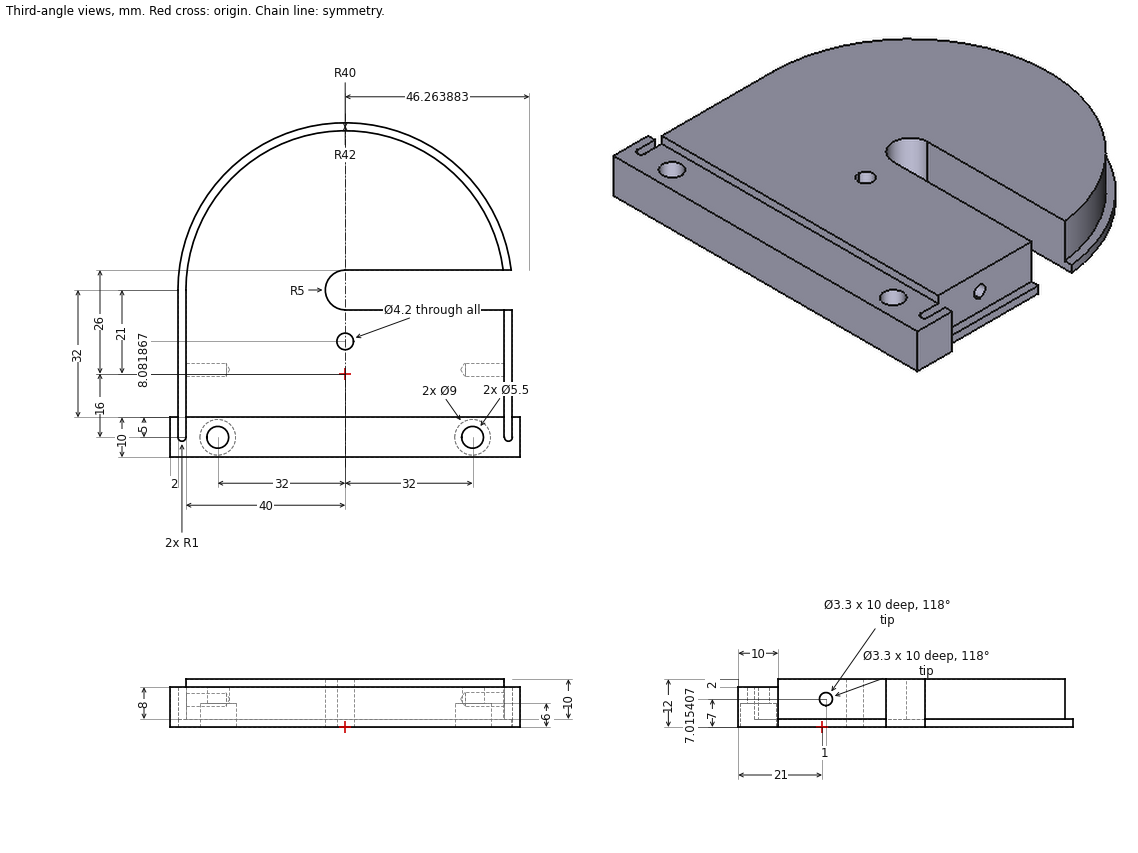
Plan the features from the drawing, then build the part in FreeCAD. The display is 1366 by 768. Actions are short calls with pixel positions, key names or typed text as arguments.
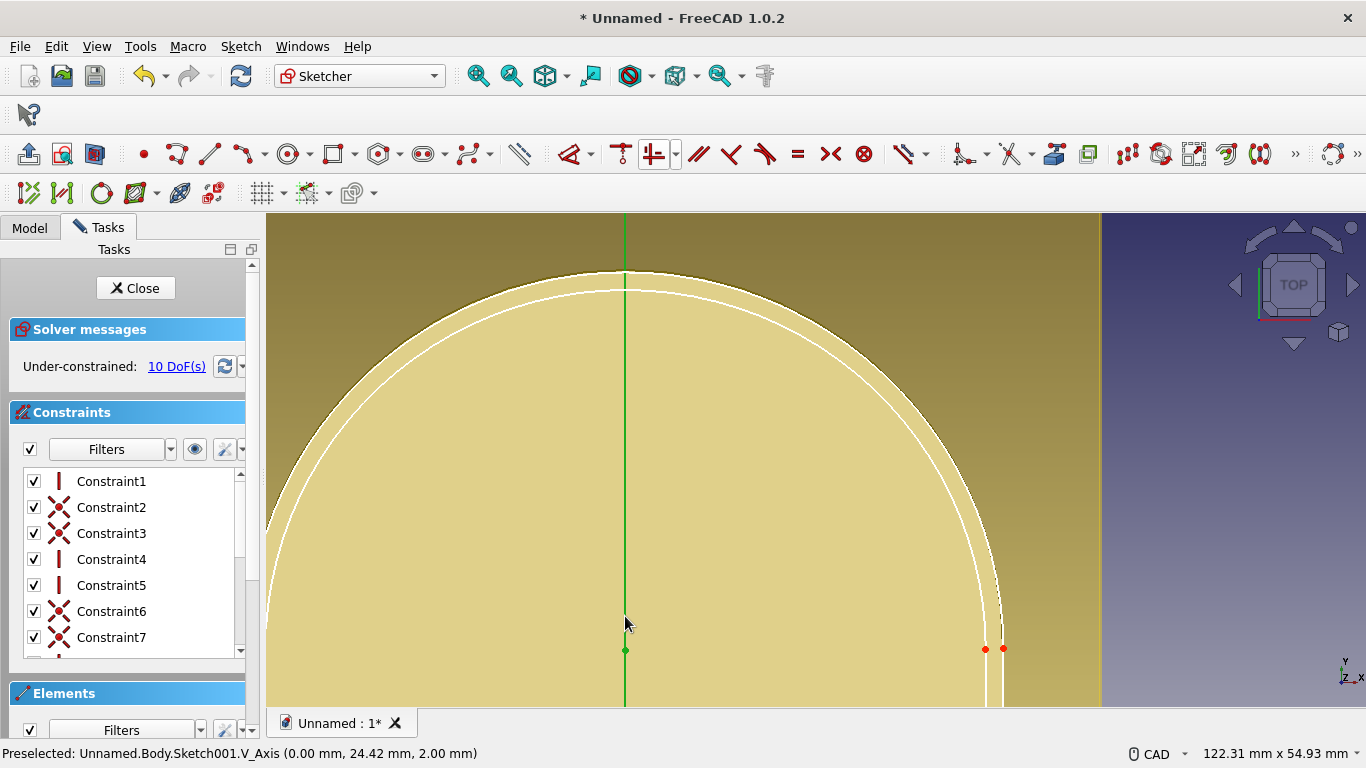
click(621, 154)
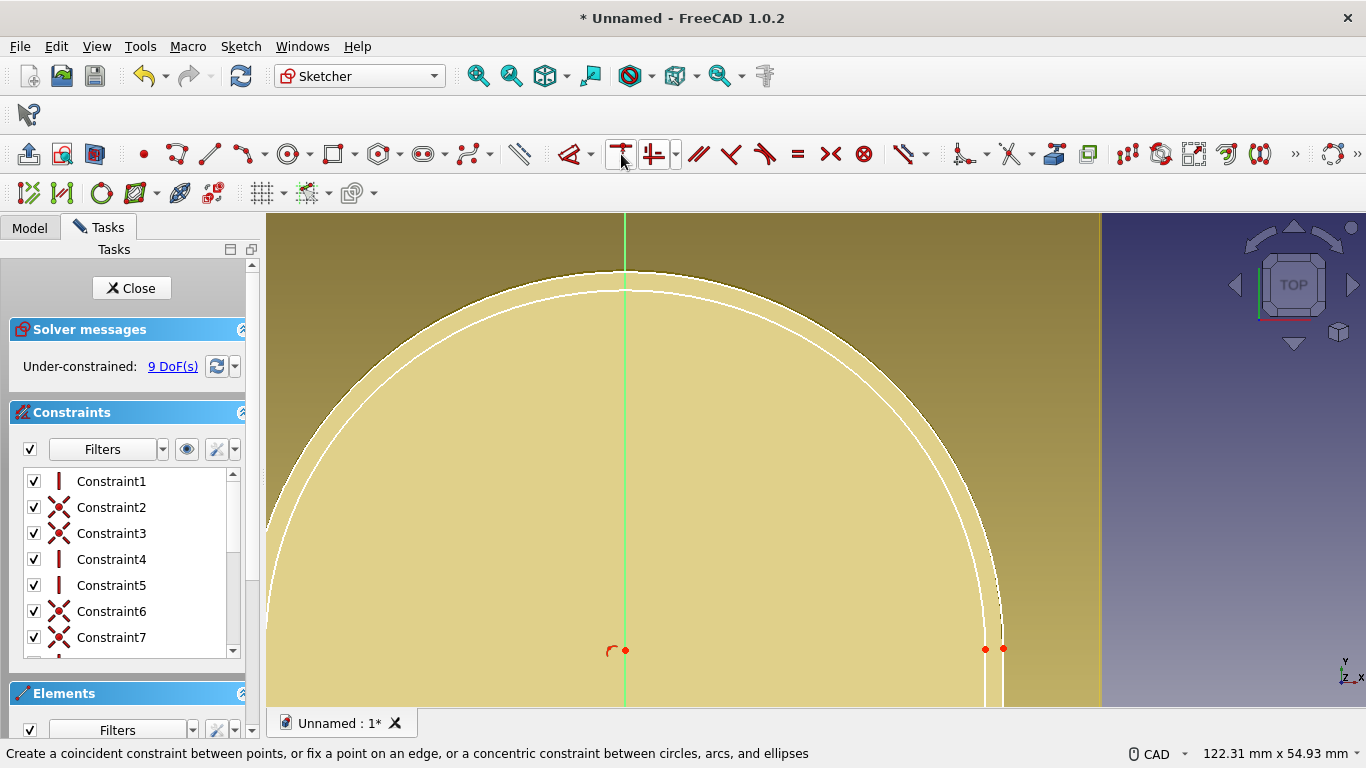
click(568, 154)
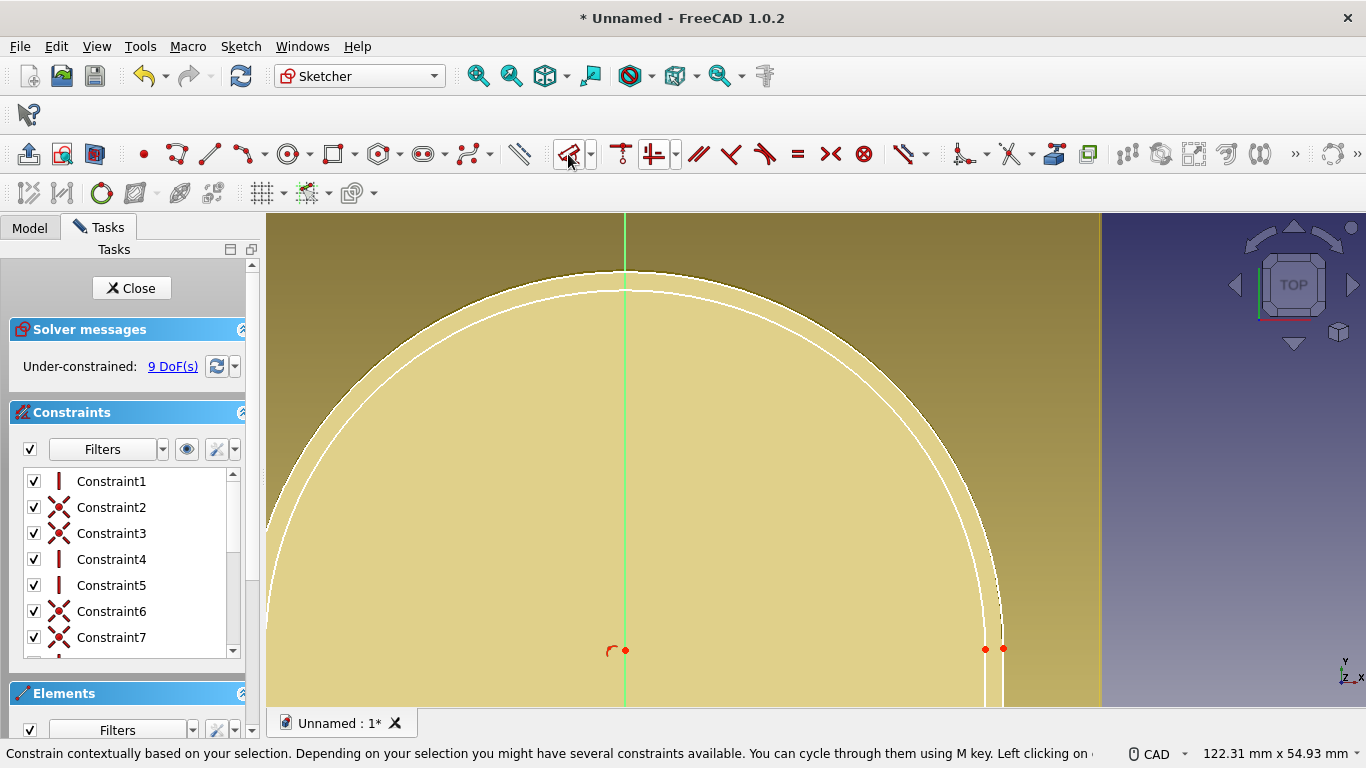
click(847, 344)
click(866, 318)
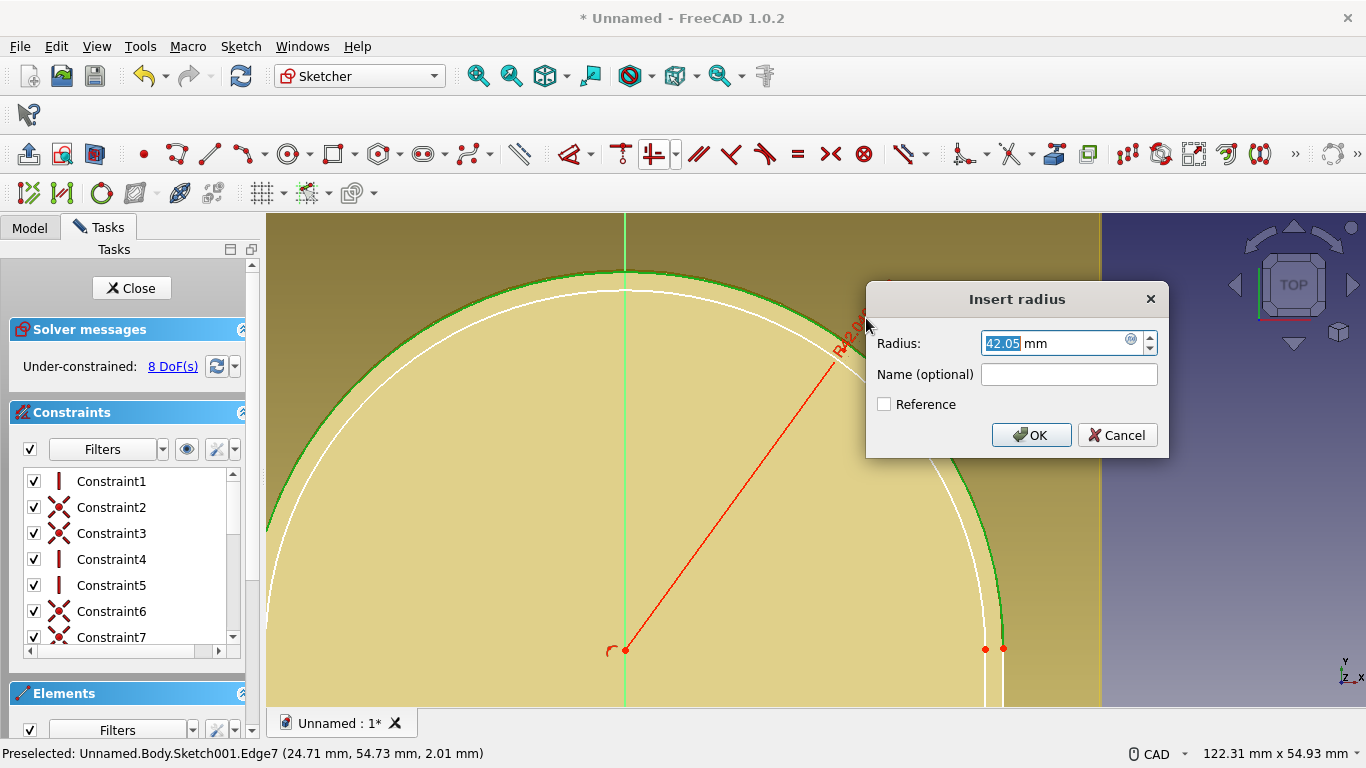
text(42)
key(Return)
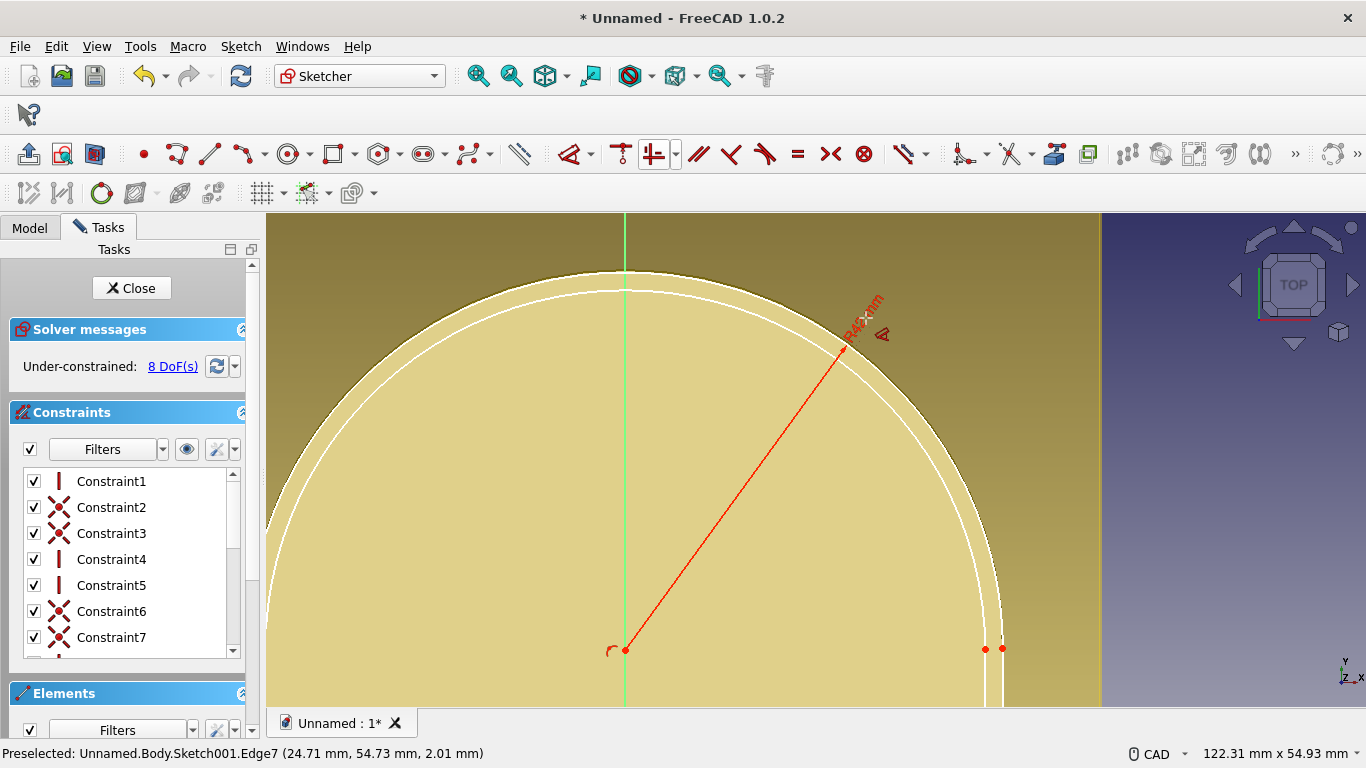
click(837, 359)
click(980, 482)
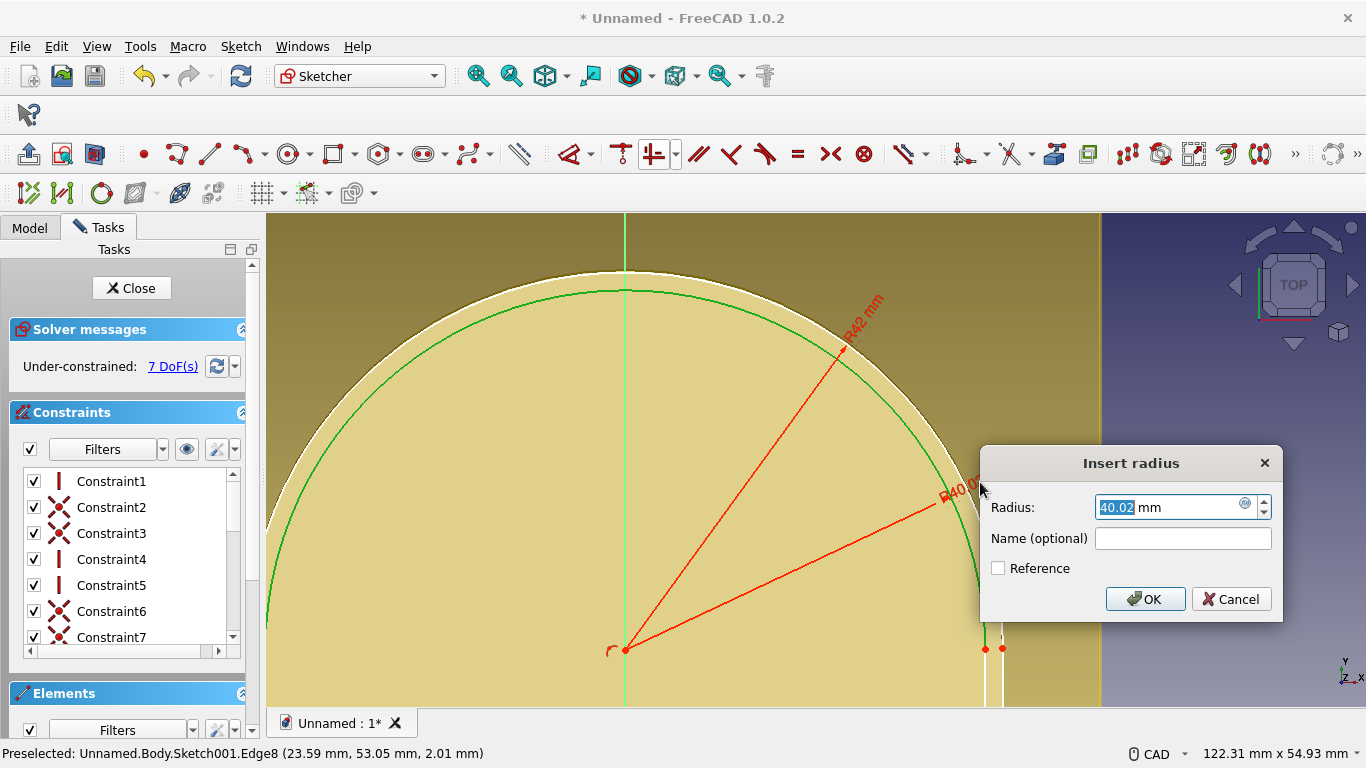
text(40)
key(Return)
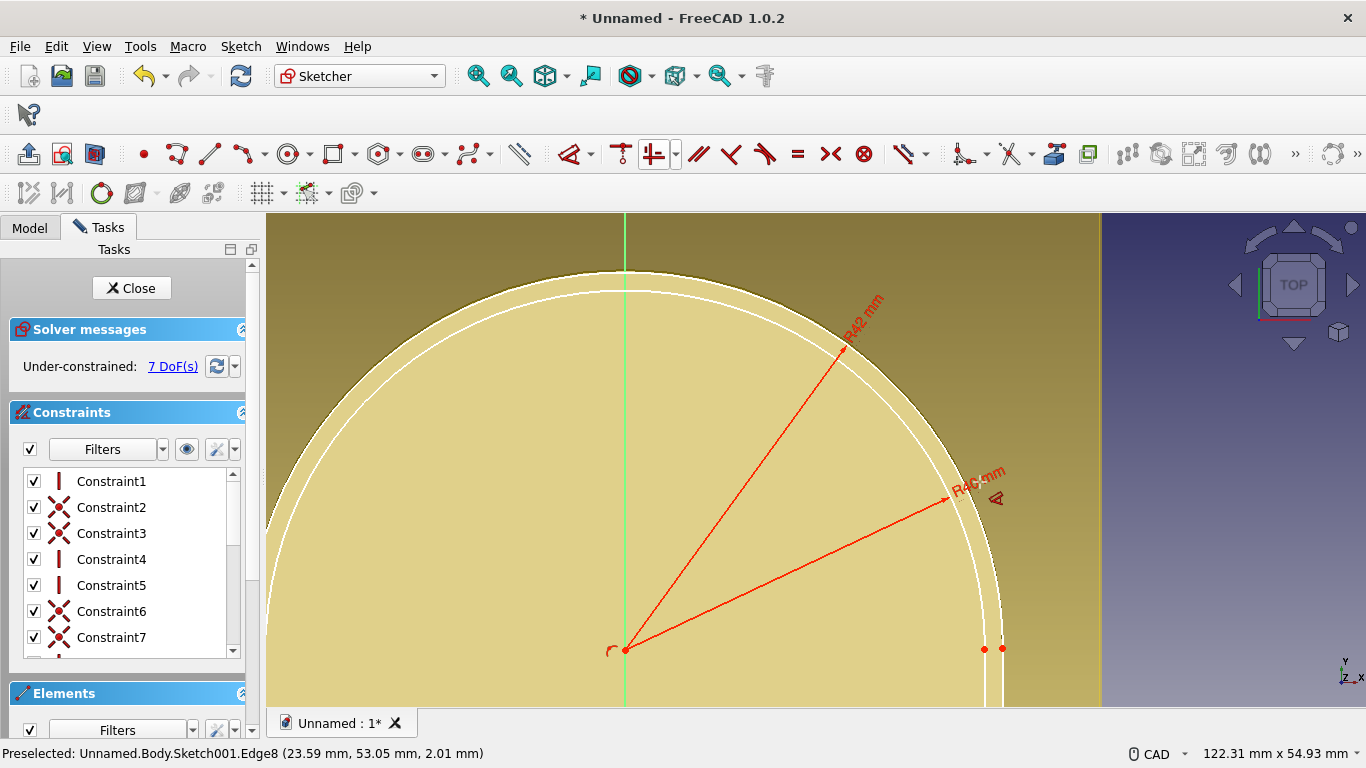
scroll(847, 344, down, 4)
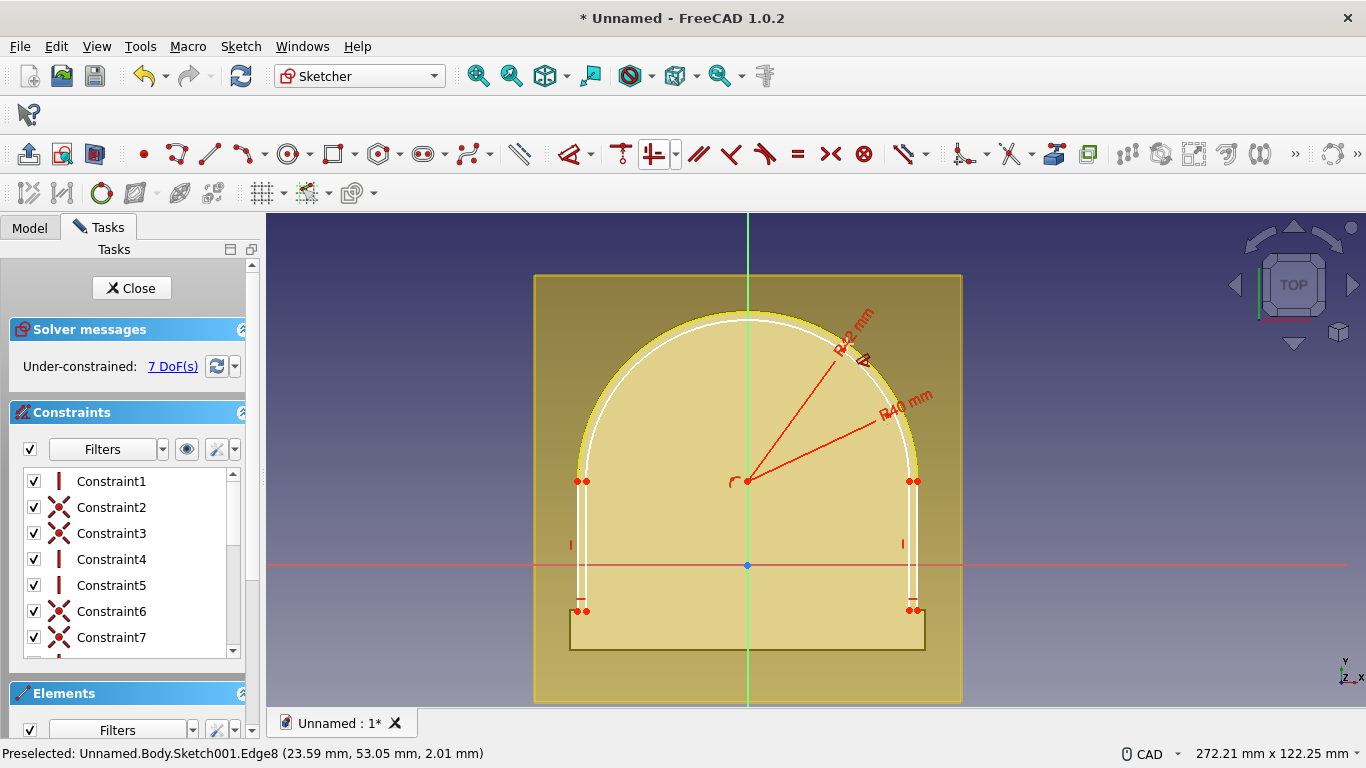
scroll(909, 520, up, 3)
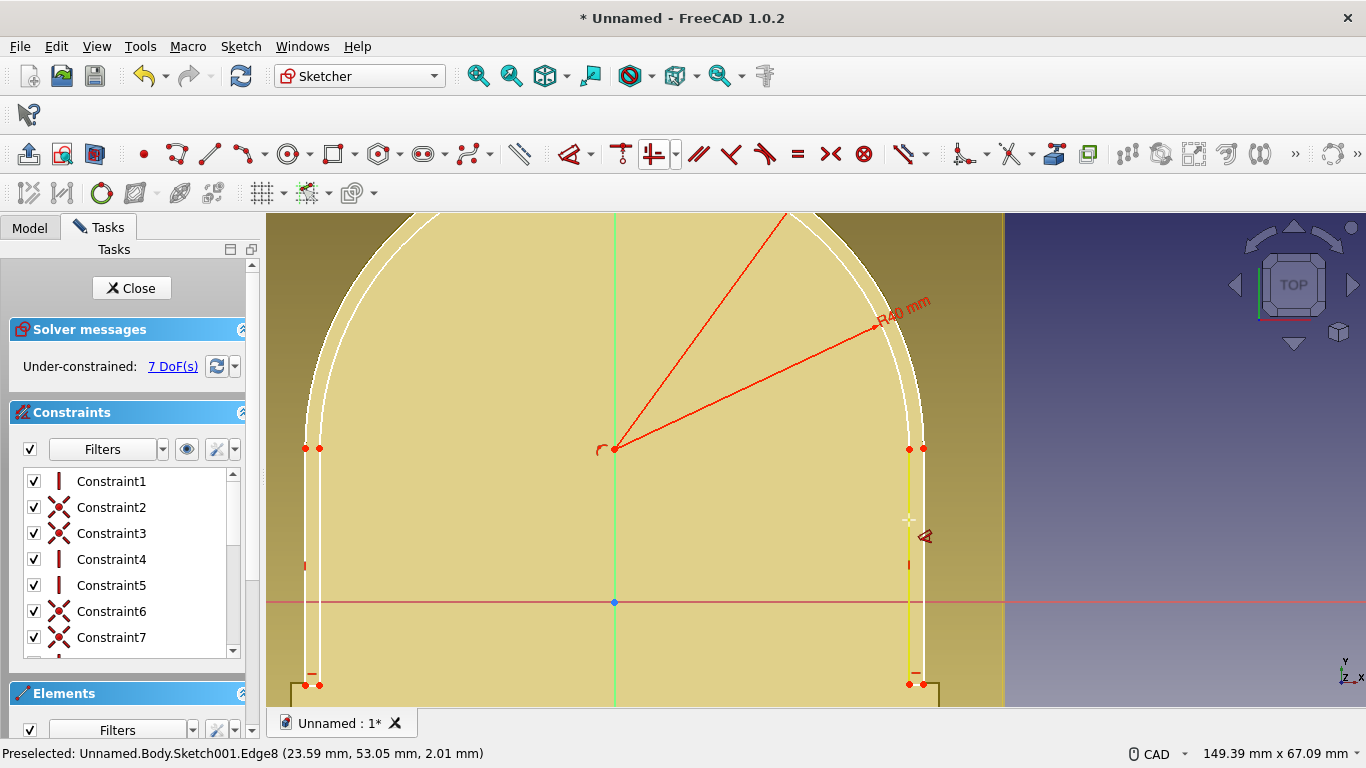
click(909, 520)
click(943, 564)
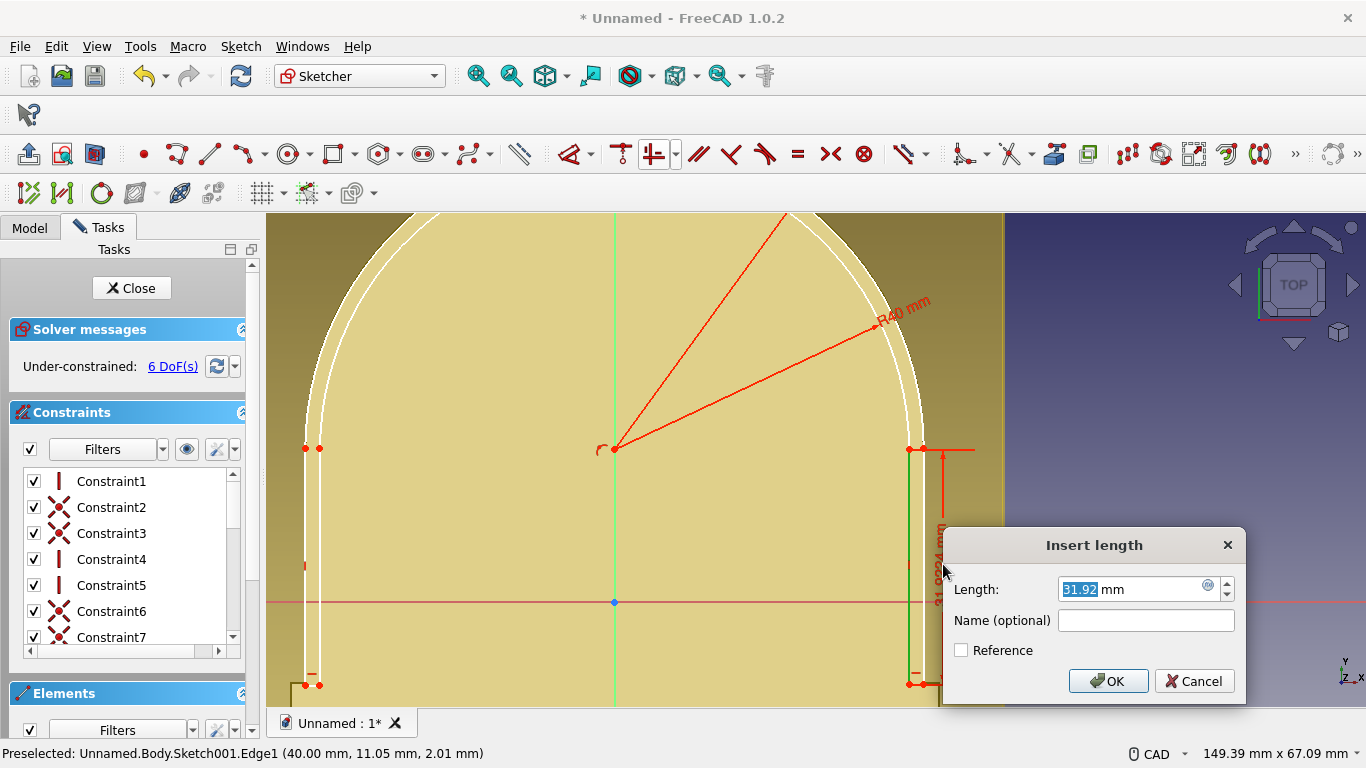
text(32)
key(Return)